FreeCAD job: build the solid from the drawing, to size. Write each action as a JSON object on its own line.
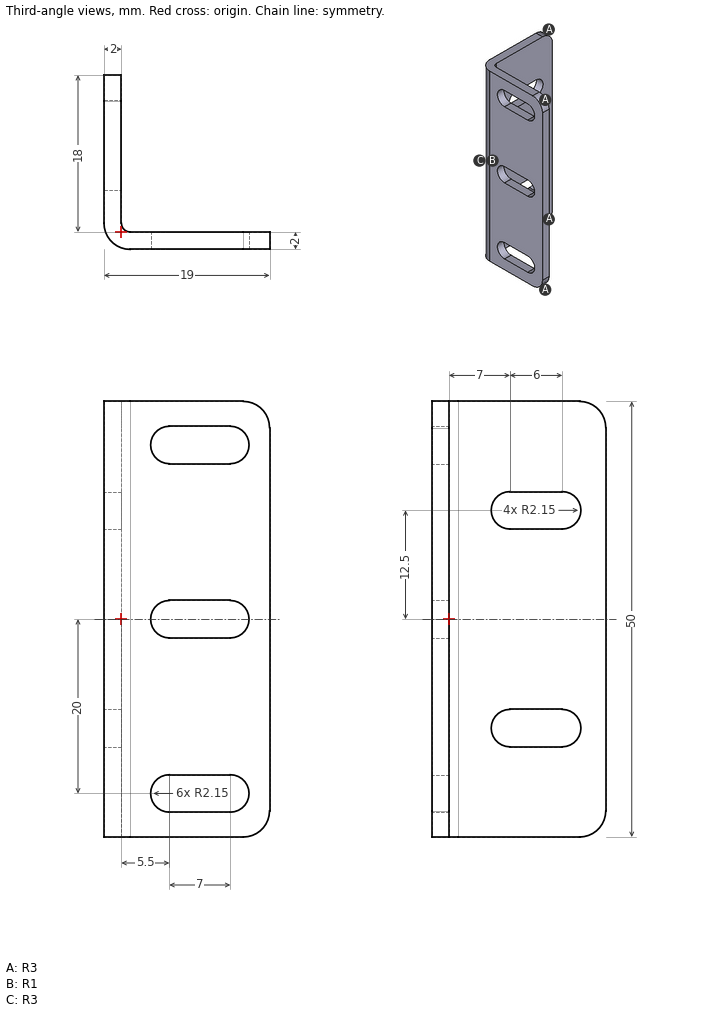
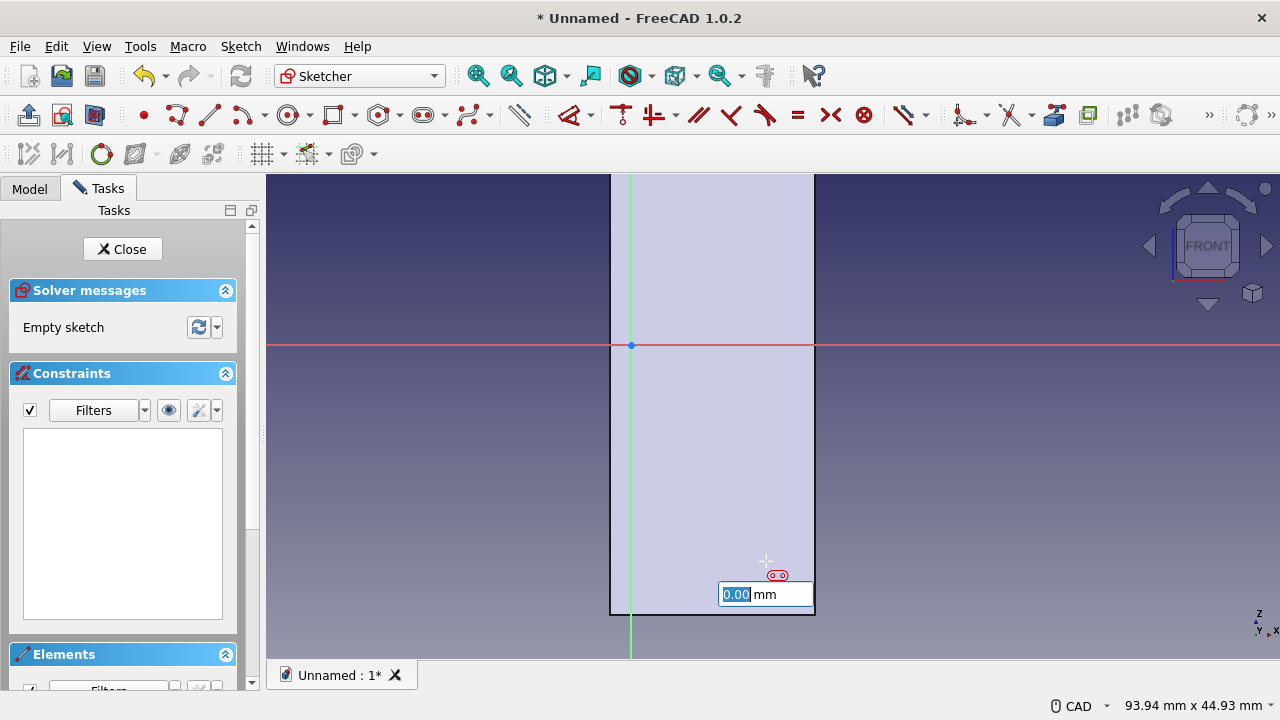
{"action": "left_click", "coordinate": [728, 584]}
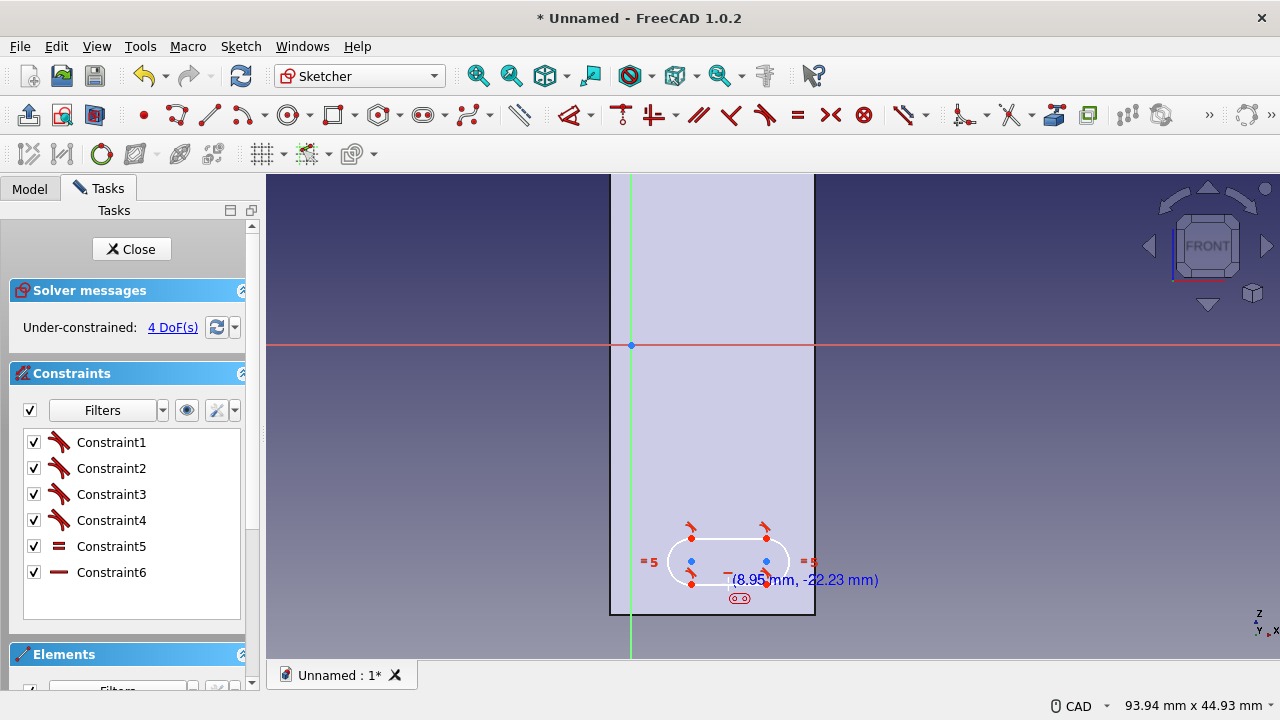
{"action": "scroll", "coordinate": [692, 562], "scroll_direction": "down", "scroll_amount": 2}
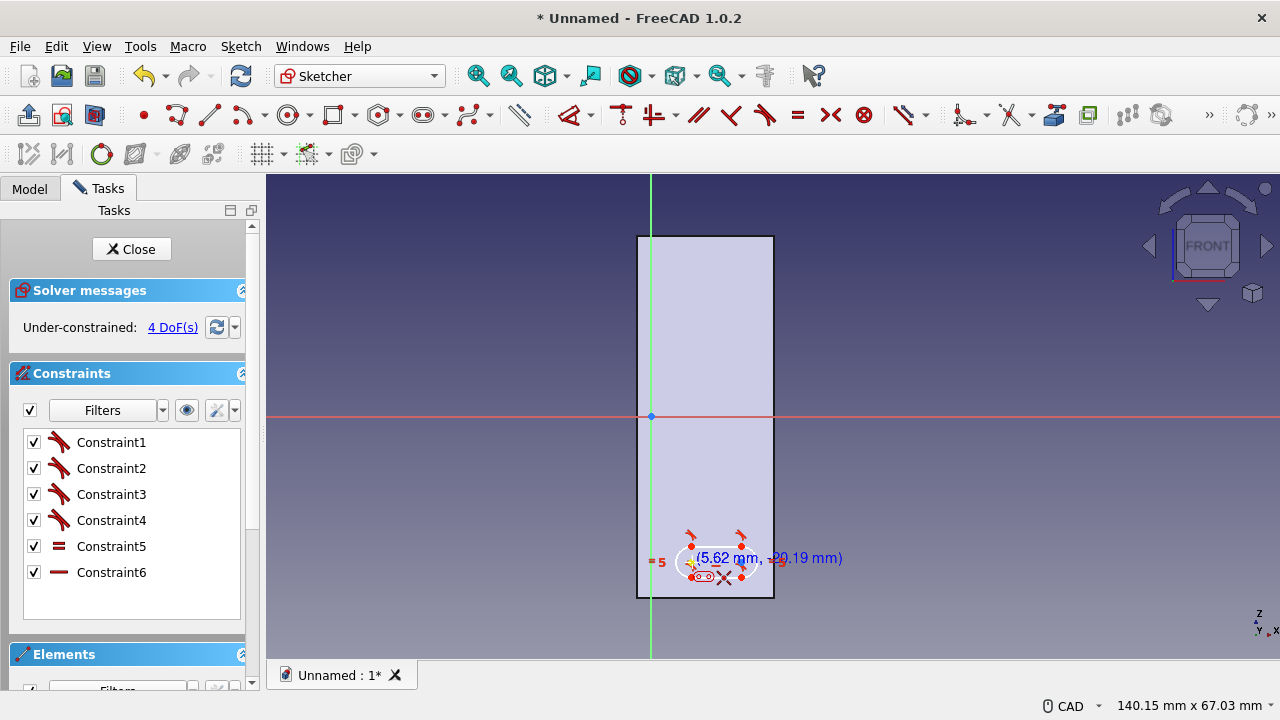
{"action": "scroll", "coordinate": [691, 272], "scroll_direction": "up", "scroll_amount": 2}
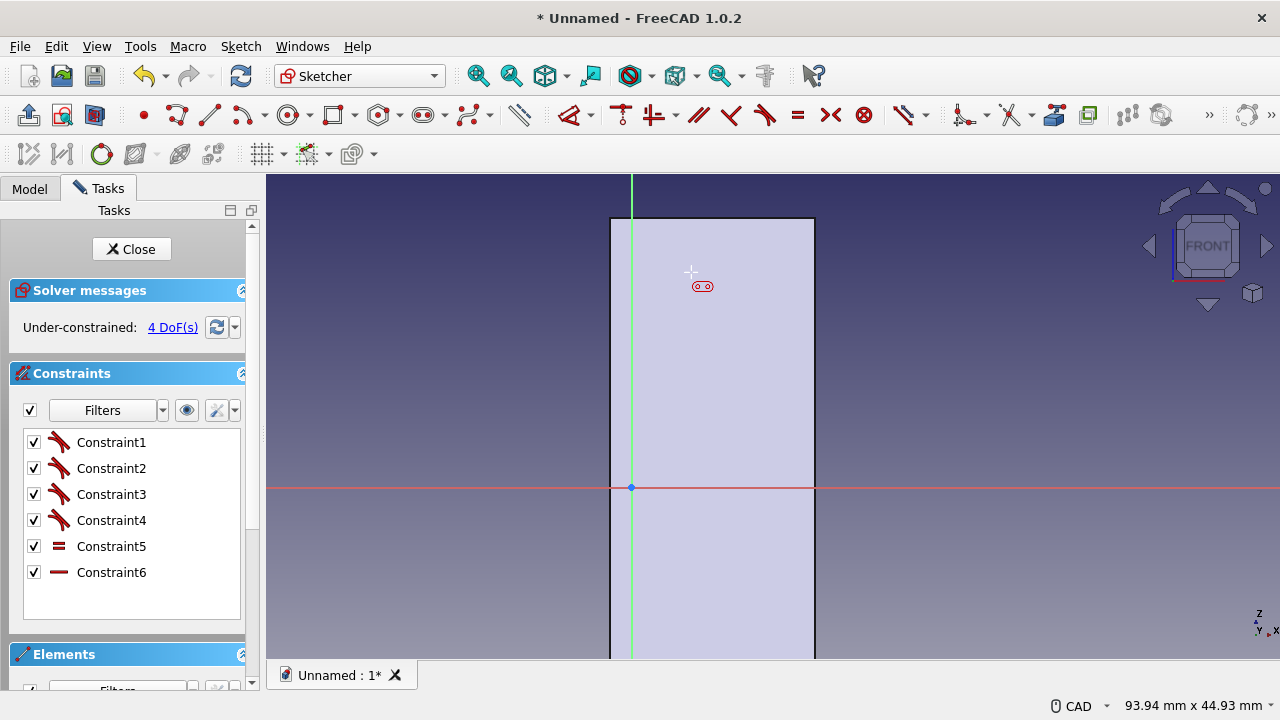
{"action": "left_click", "coordinate": [691, 272]}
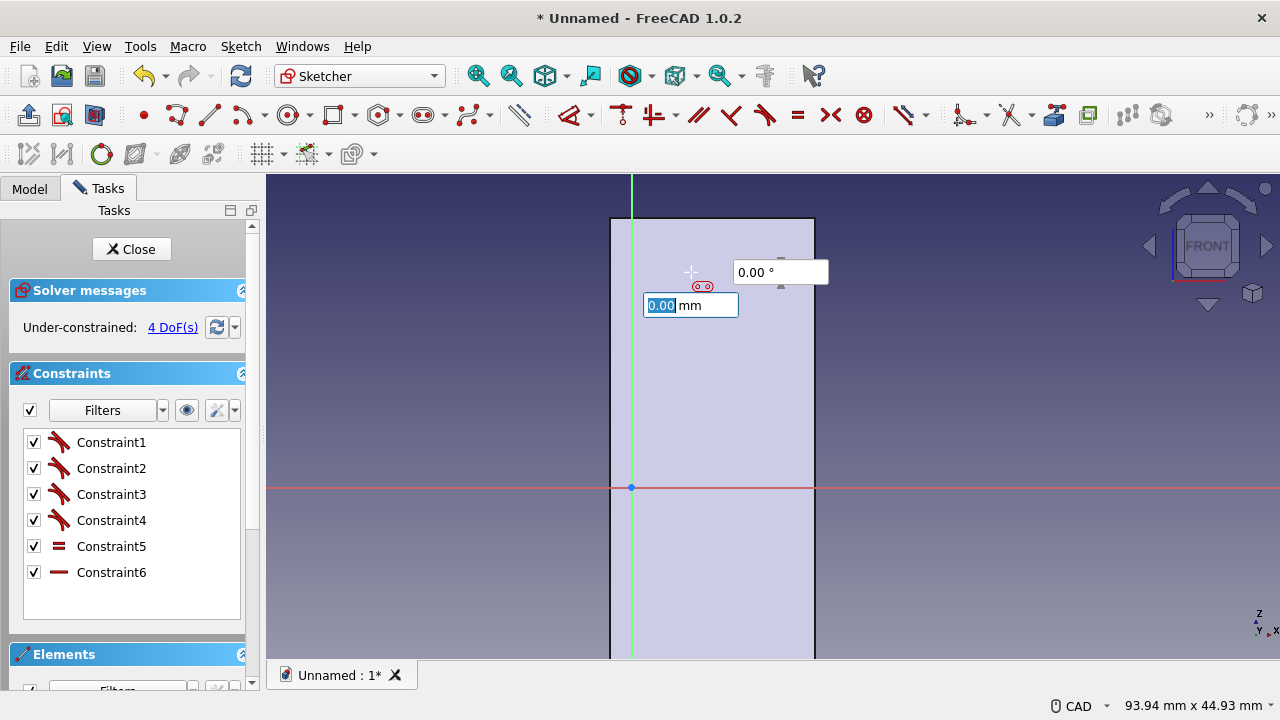
{"action": "left_click", "coordinate": [767, 272]}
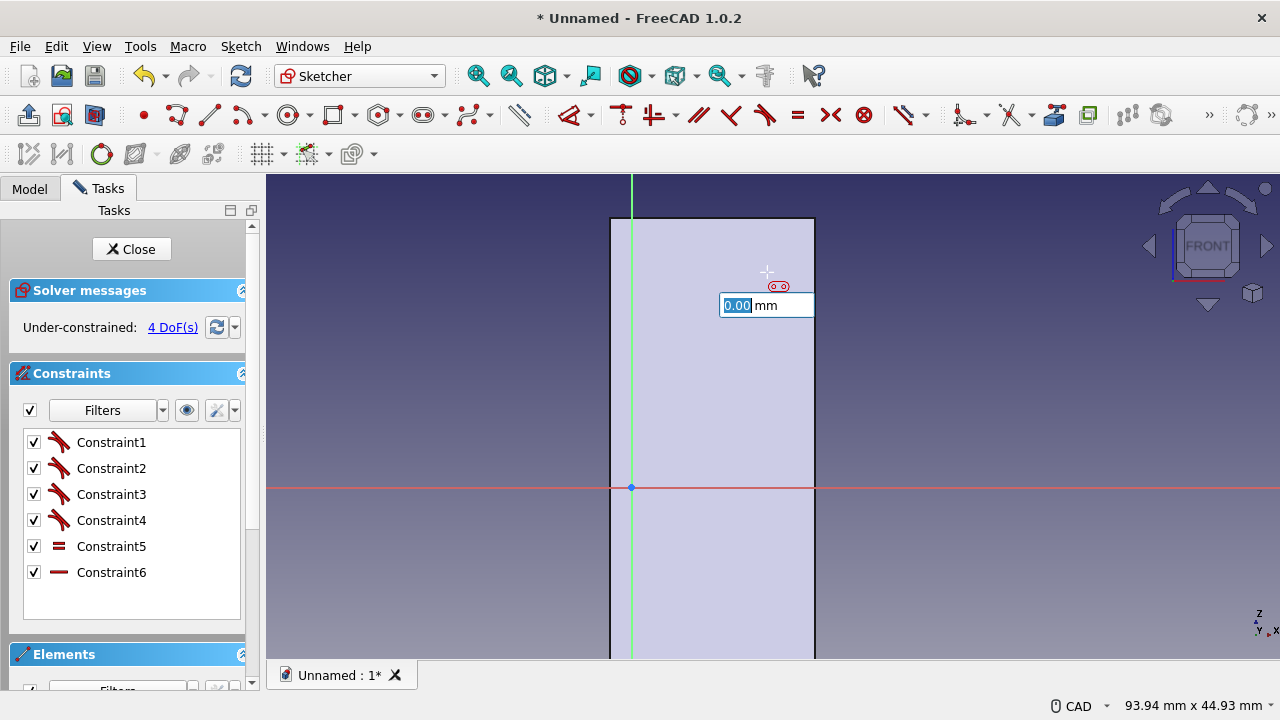
{"action": "left_click", "coordinate": [729, 249]}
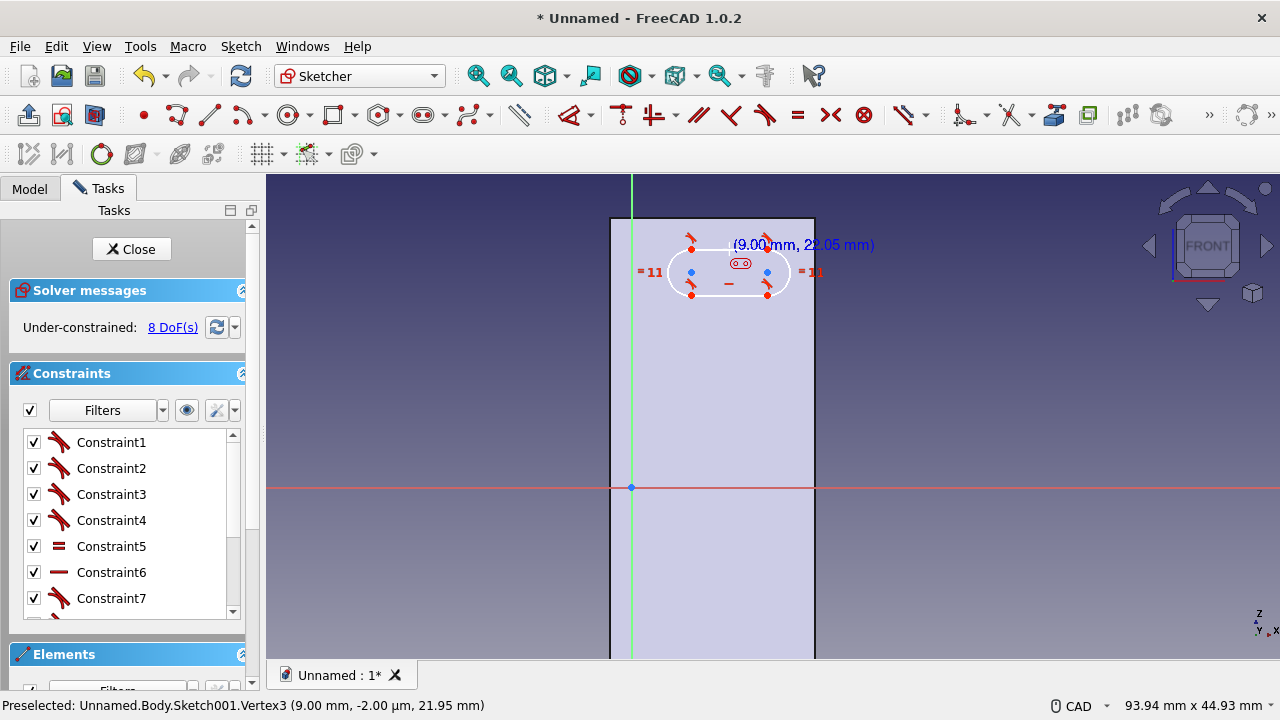
{"action": "left_click", "coordinate": [691, 488]}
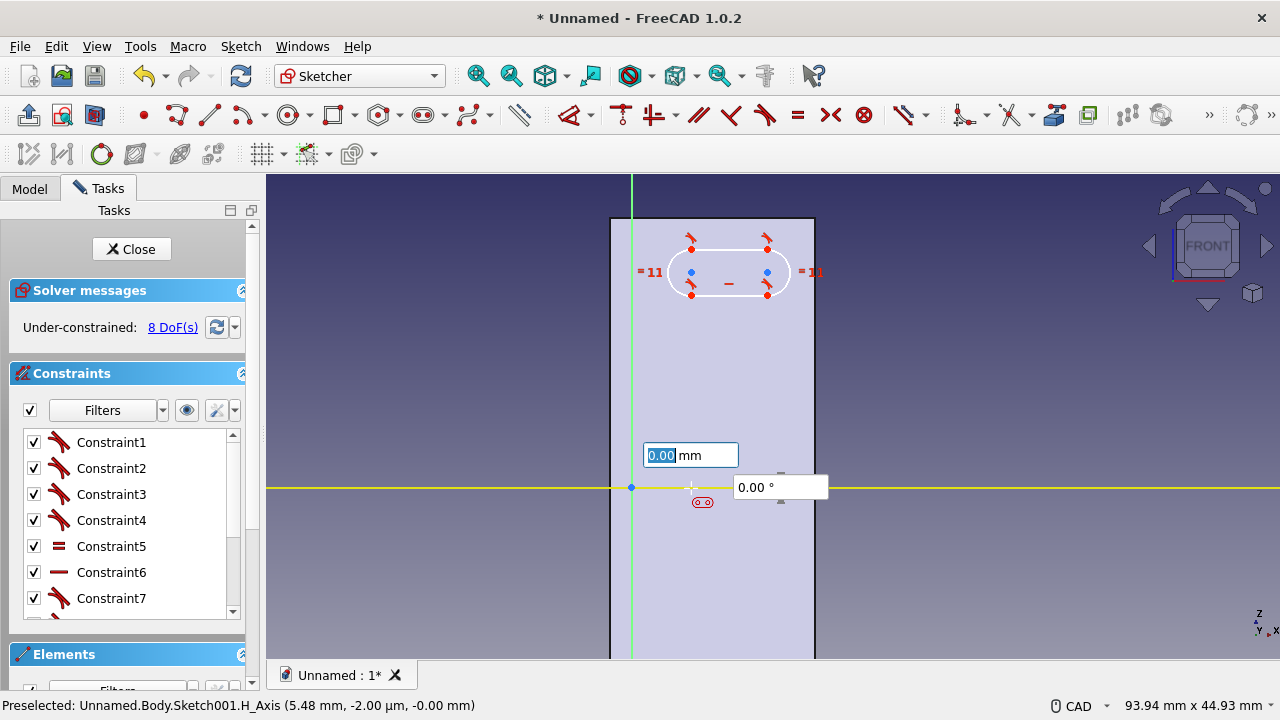
{"action": "left_click", "coordinate": [767, 479]}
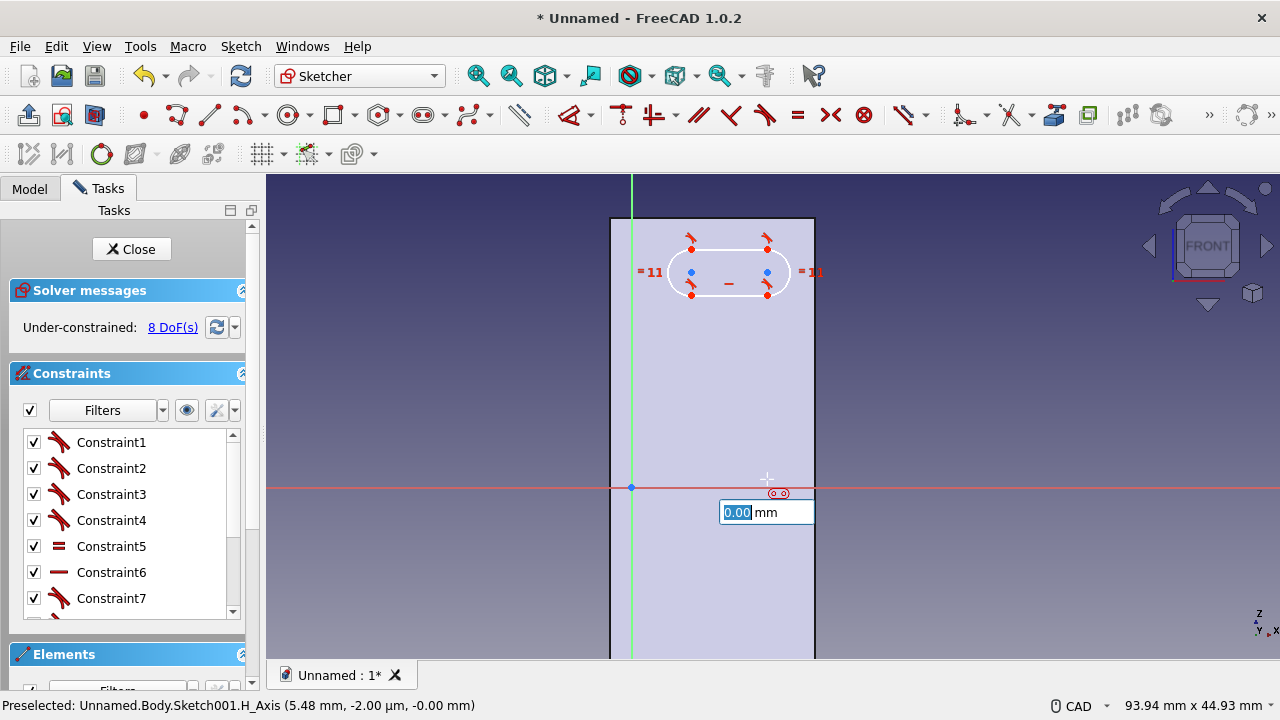
{"action": "left_click", "coordinate": [729, 511]}
{"action": "key", "text": "Escape"}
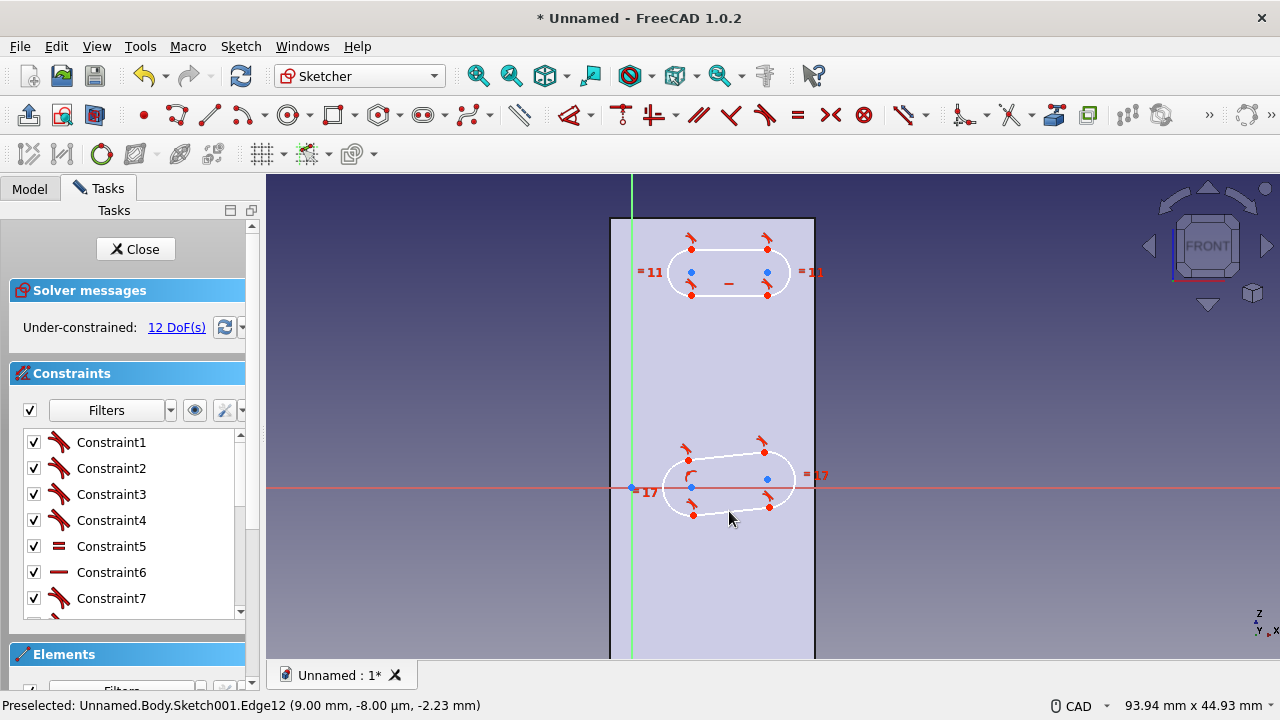
{"action": "left_click", "coordinate": [711, 458]}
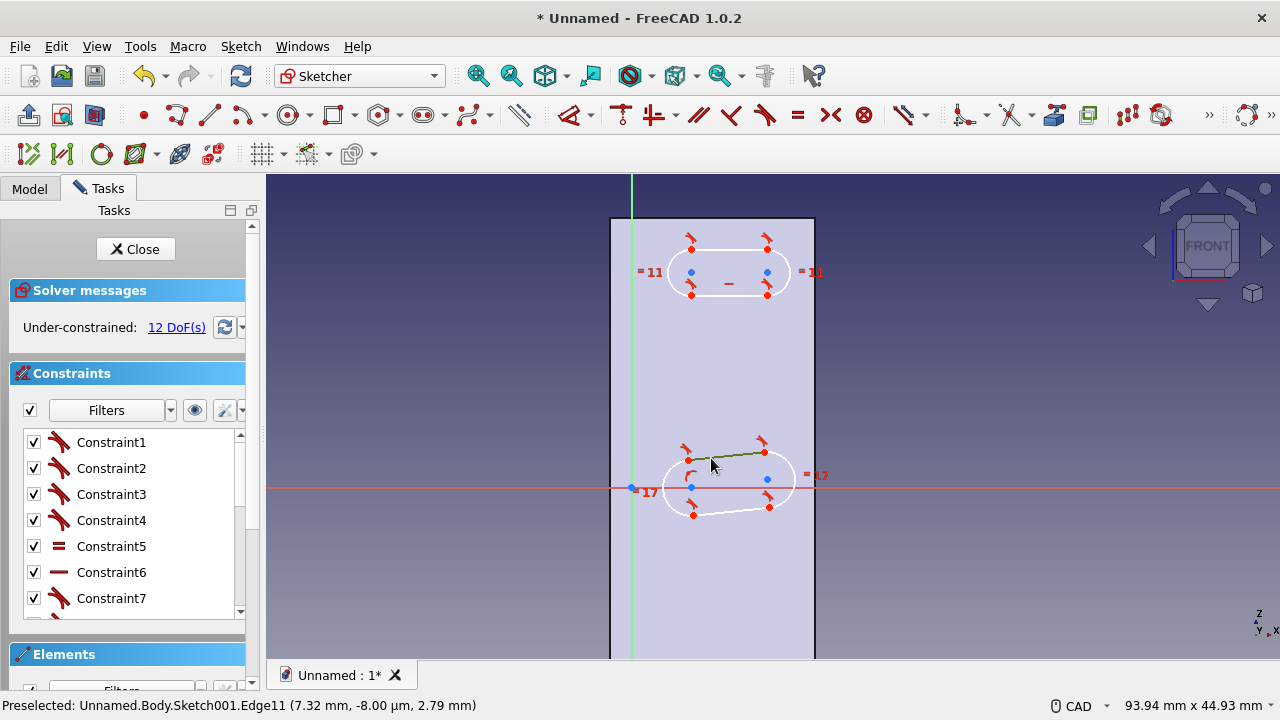
{"action": "left_click", "coordinate": [676, 116]}